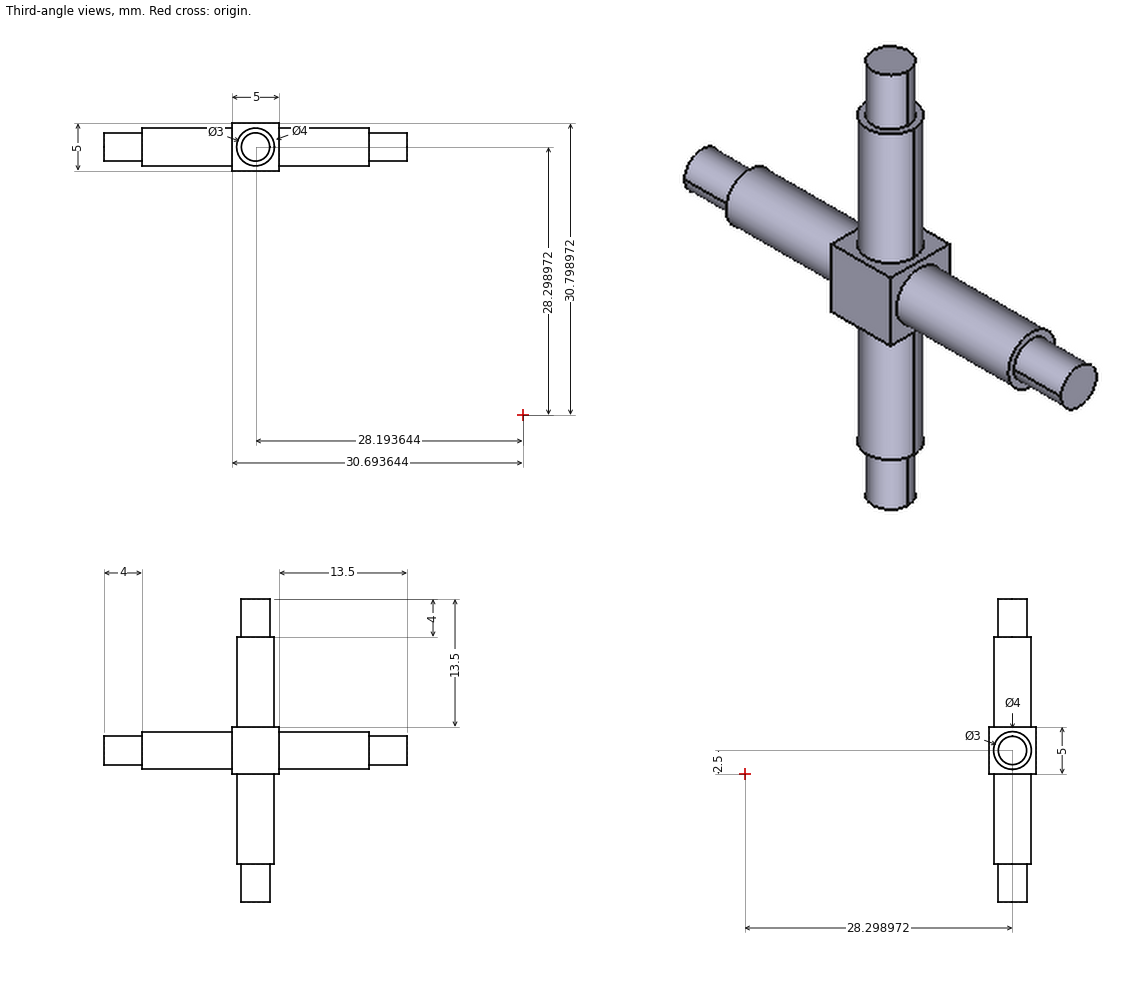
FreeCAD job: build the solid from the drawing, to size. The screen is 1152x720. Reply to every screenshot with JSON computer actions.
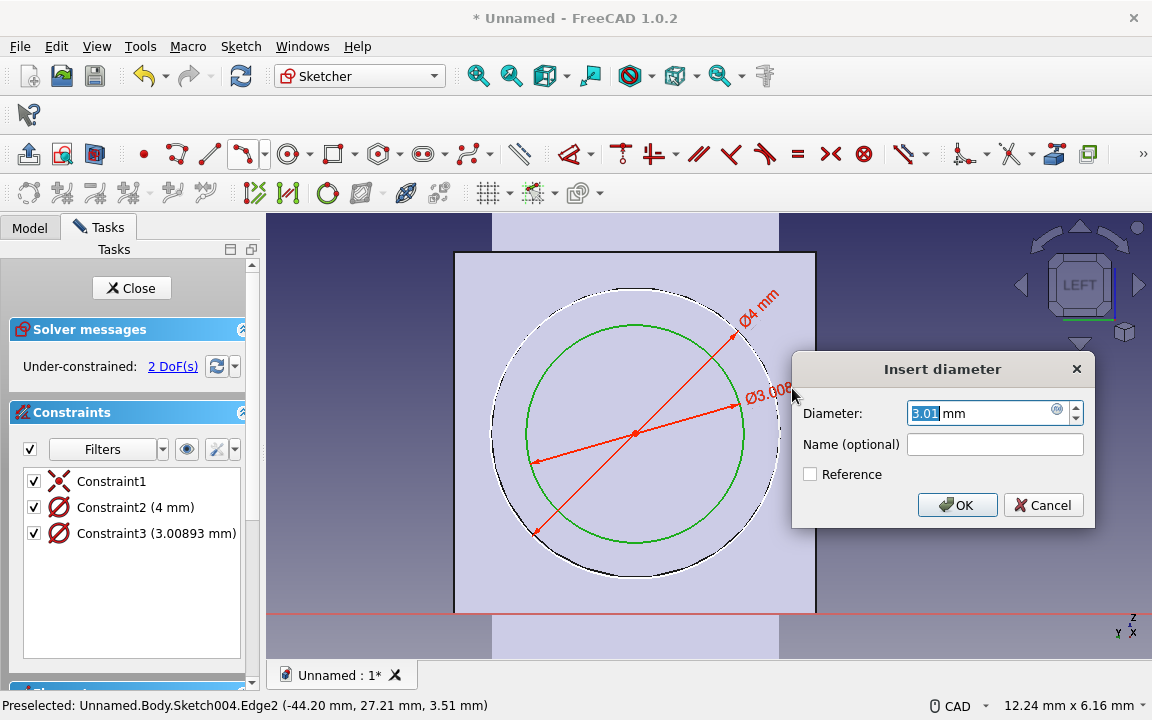
{"action": "type", "text": "3"}
{"action": "key", "text": "Return"}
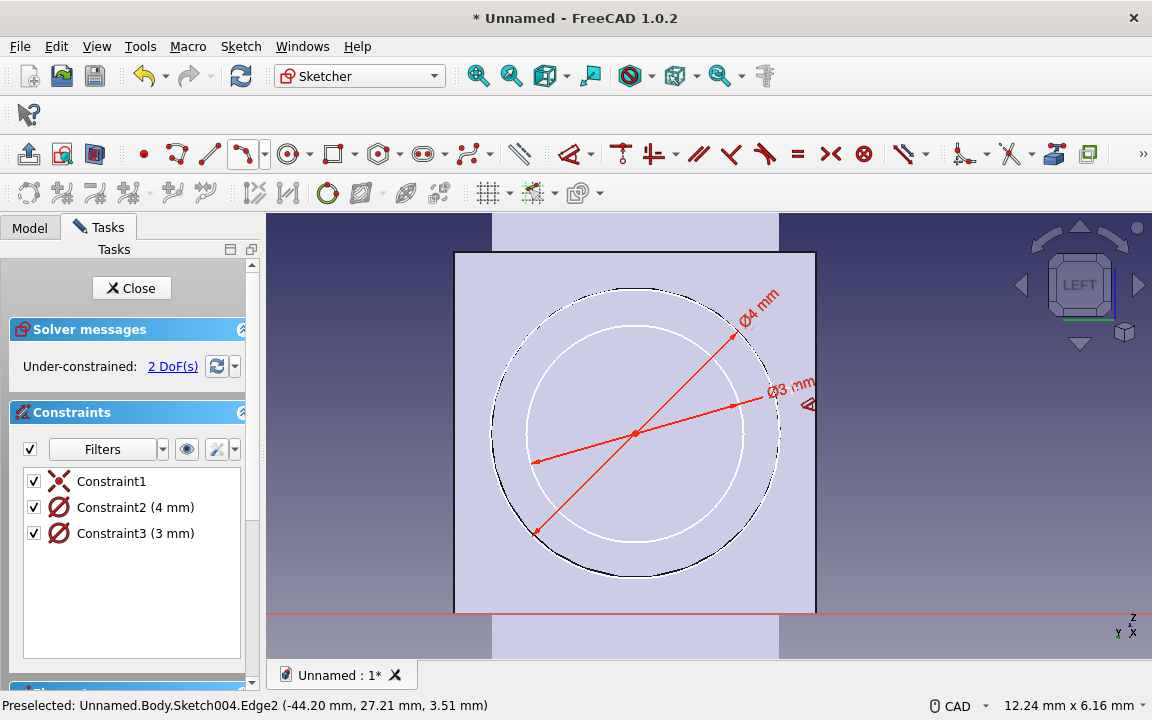
{"action": "left_click", "coordinate": [635, 434]}
{"action": "left_click", "coordinate": [601, 483]}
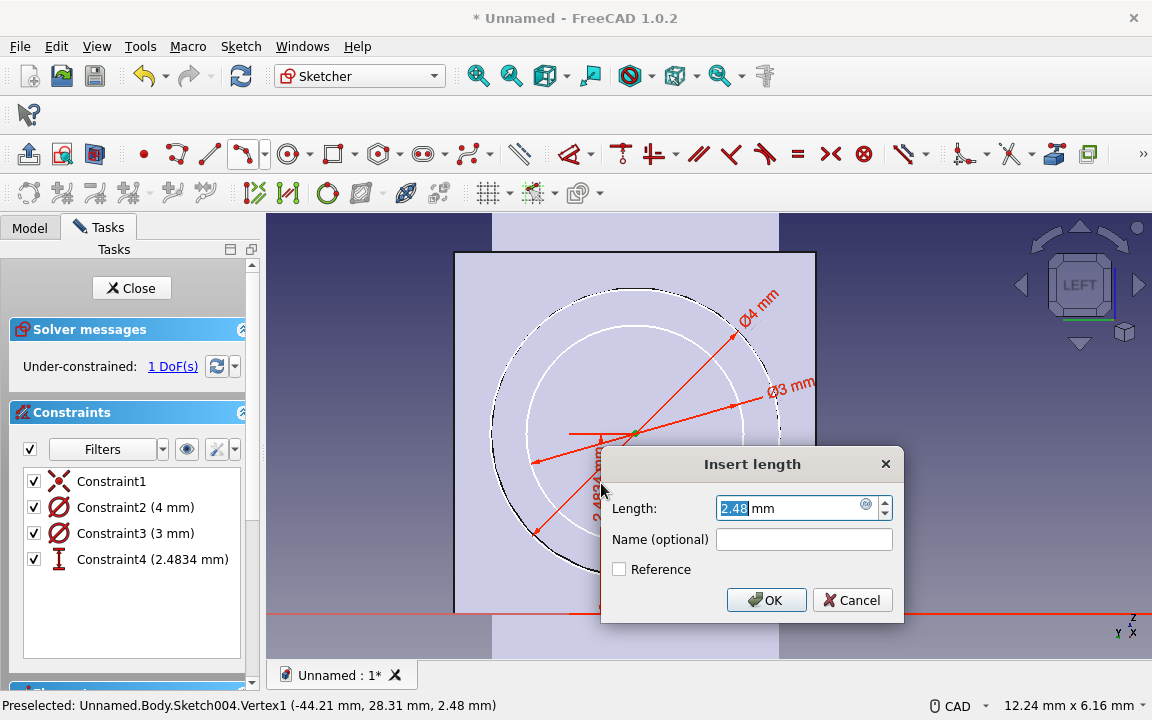
{"action": "type", "text": "2.5"}
{"action": "key", "text": "Return"}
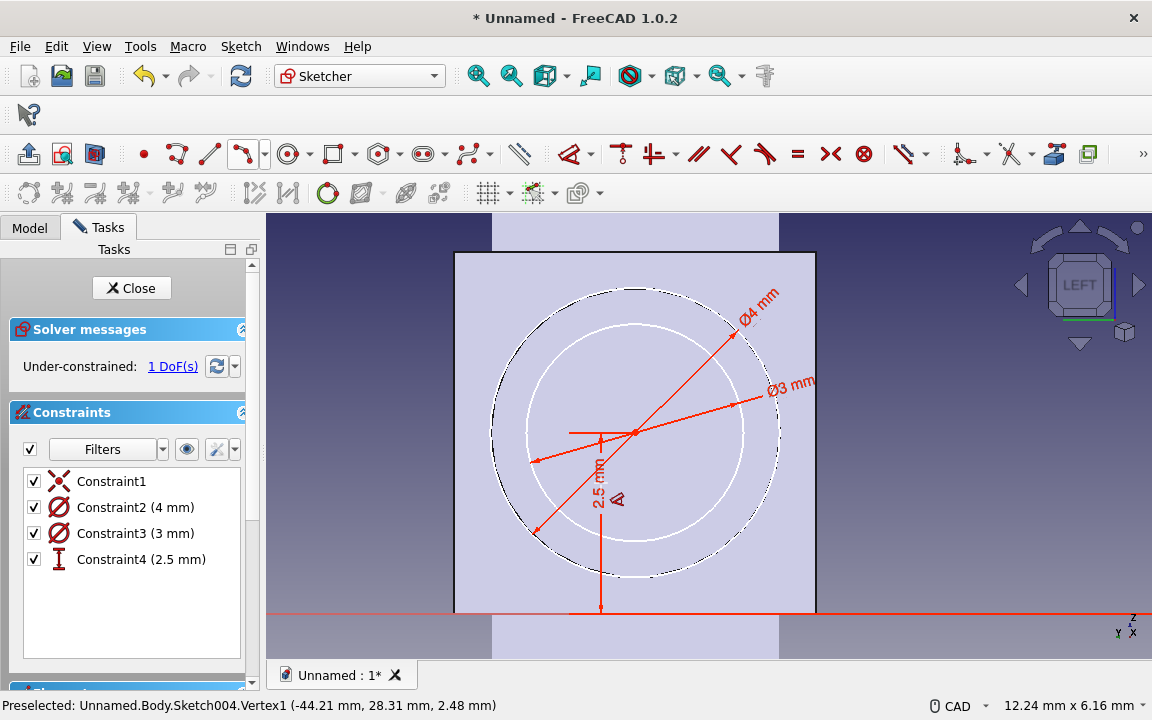
{"action": "left_click", "coordinate": [635, 433]}
{"action": "left_click", "coordinate": [892, 399]}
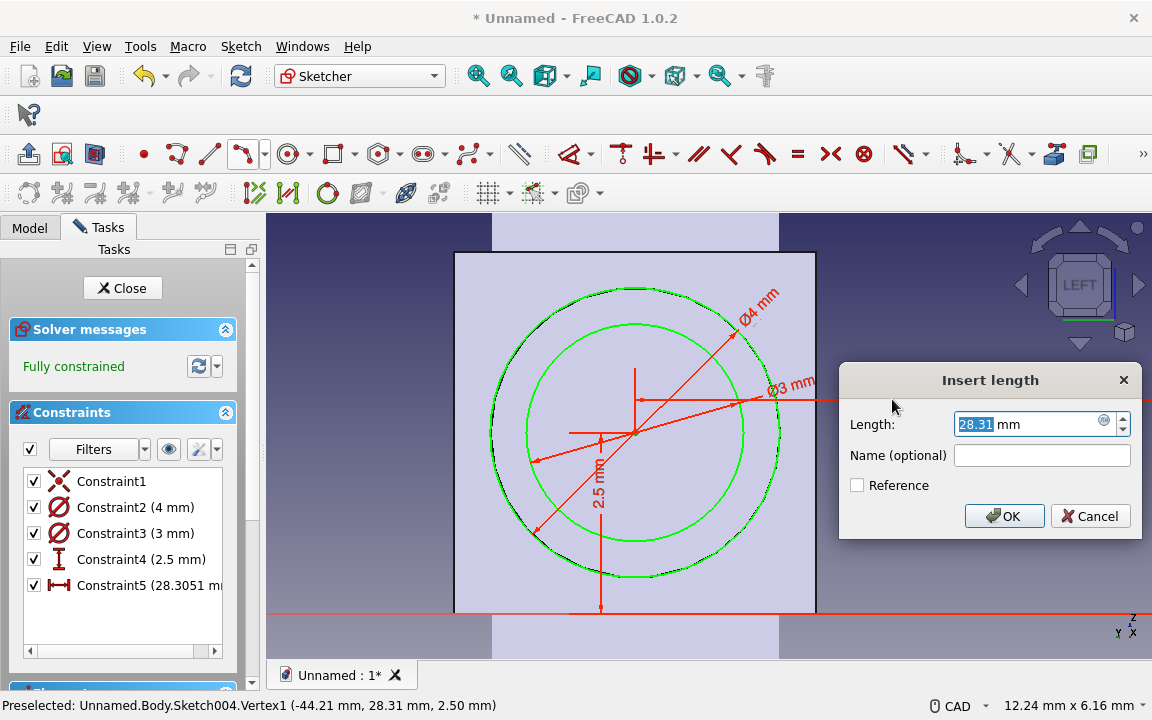
{"action": "type", "text": "28.298972"}
{"action": "key", "text": "Return"}
{"action": "key", "text": "Escape"}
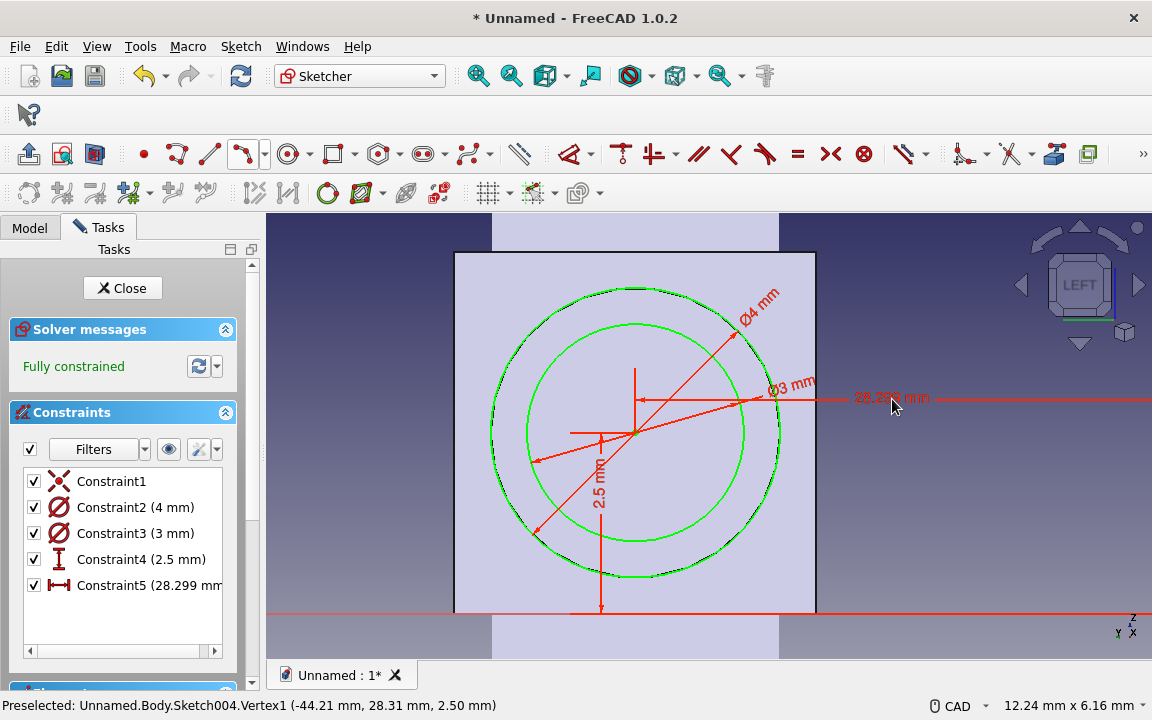
{"action": "left_click", "coordinate": [123, 288]}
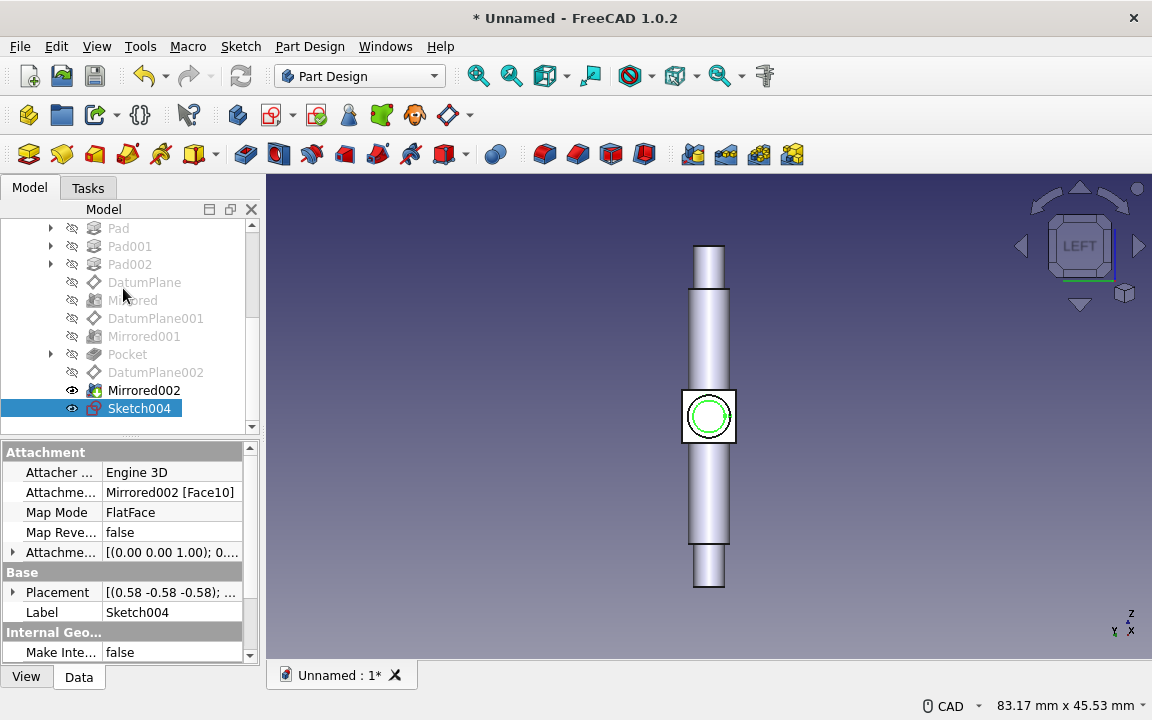
{"action": "left_click", "coordinate": [246, 154]}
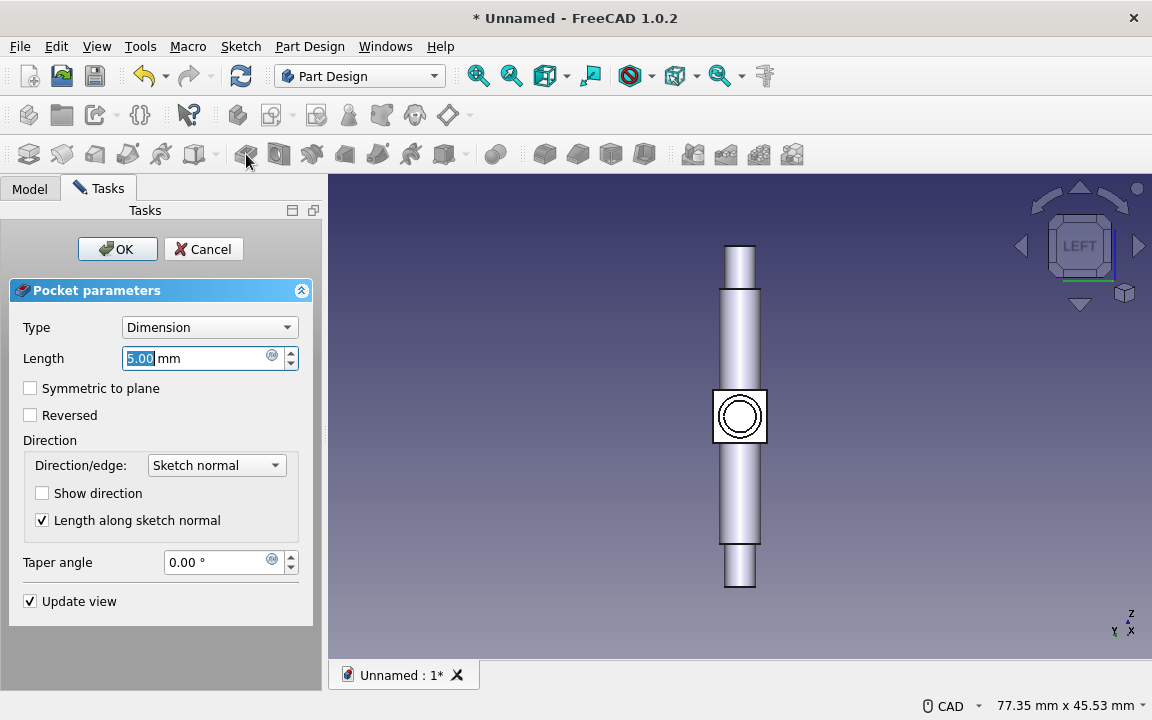
{"action": "type", "text": "4"}
{"action": "key", "text": "Tab"}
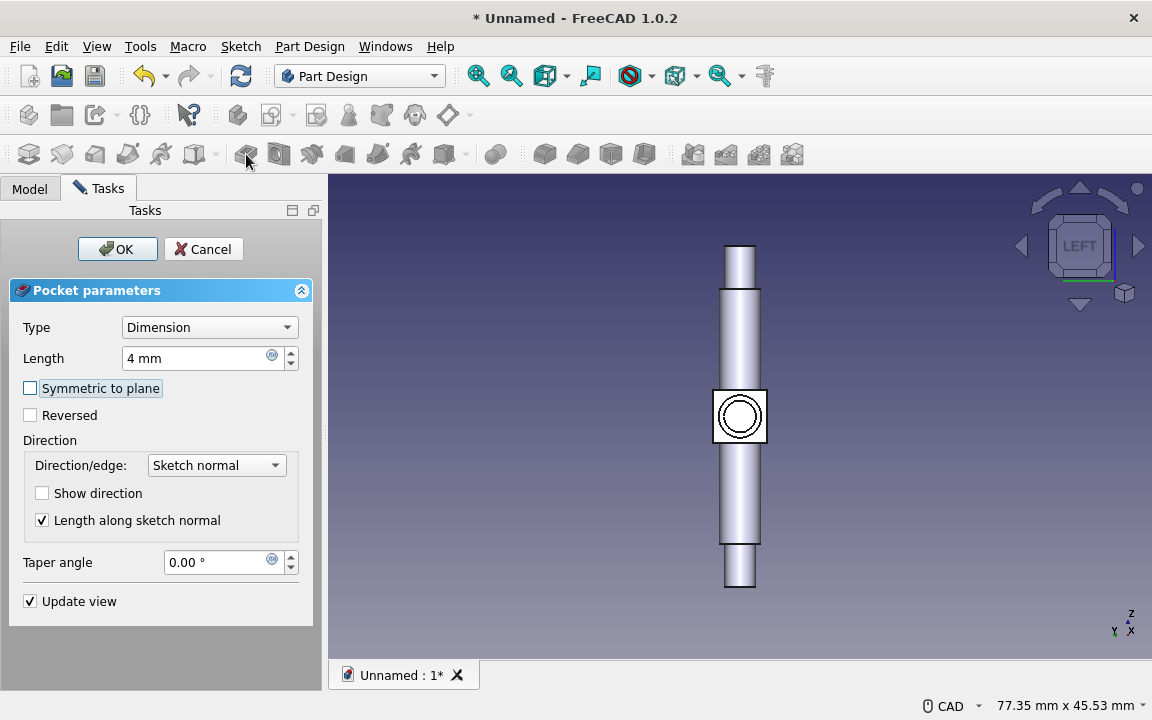
{"action": "left_click", "coordinate": [118, 249]}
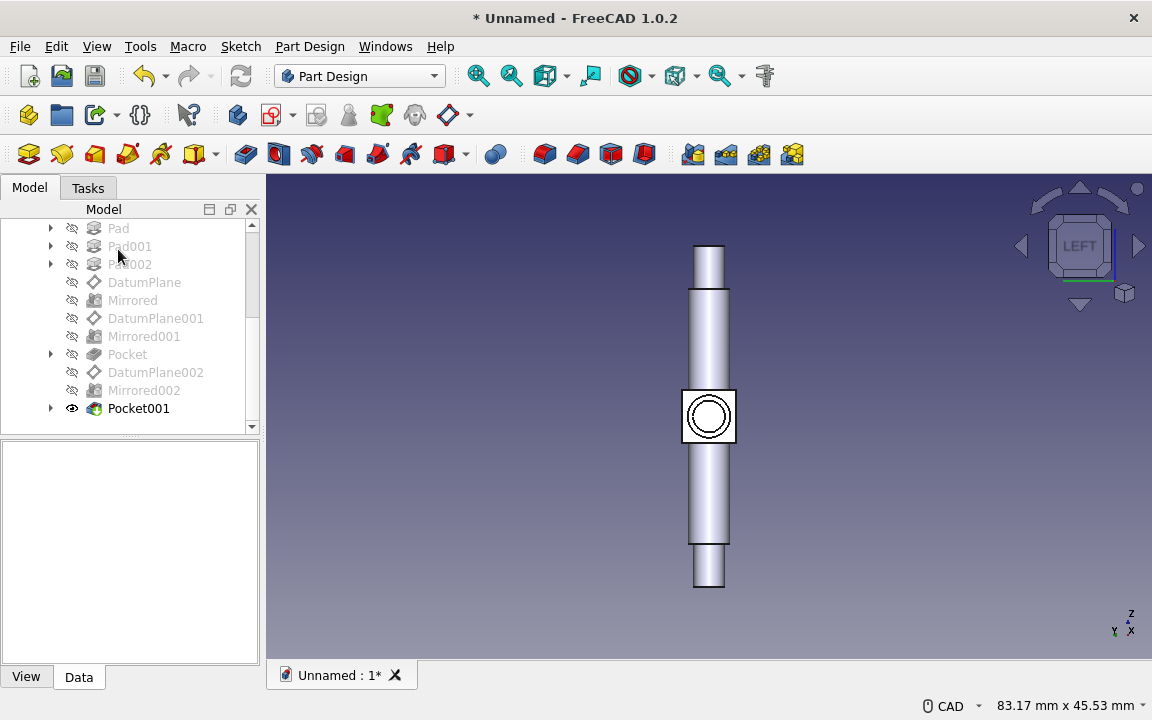
{"action": "scroll", "coordinate": [141, 314], "scroll_direction": "down", "scroll_amount": 3}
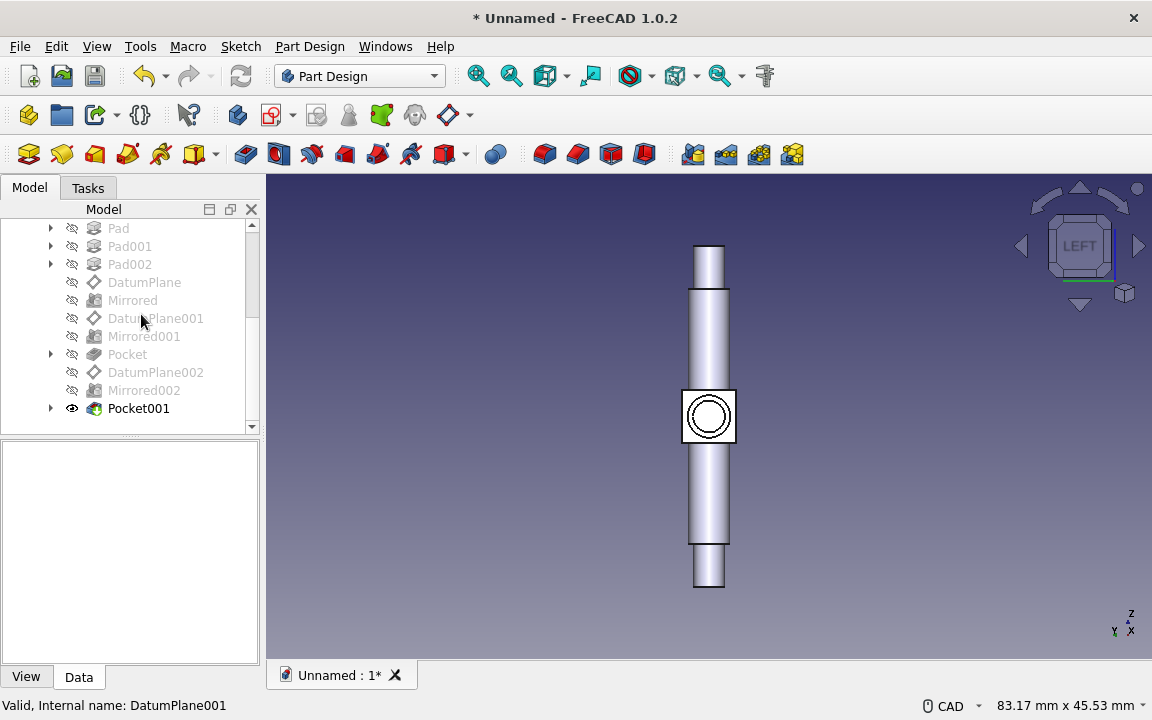
{"action": "scroll", "coordinate": [141, 314], "scroll_direction": "up", "scroll_amount": 15}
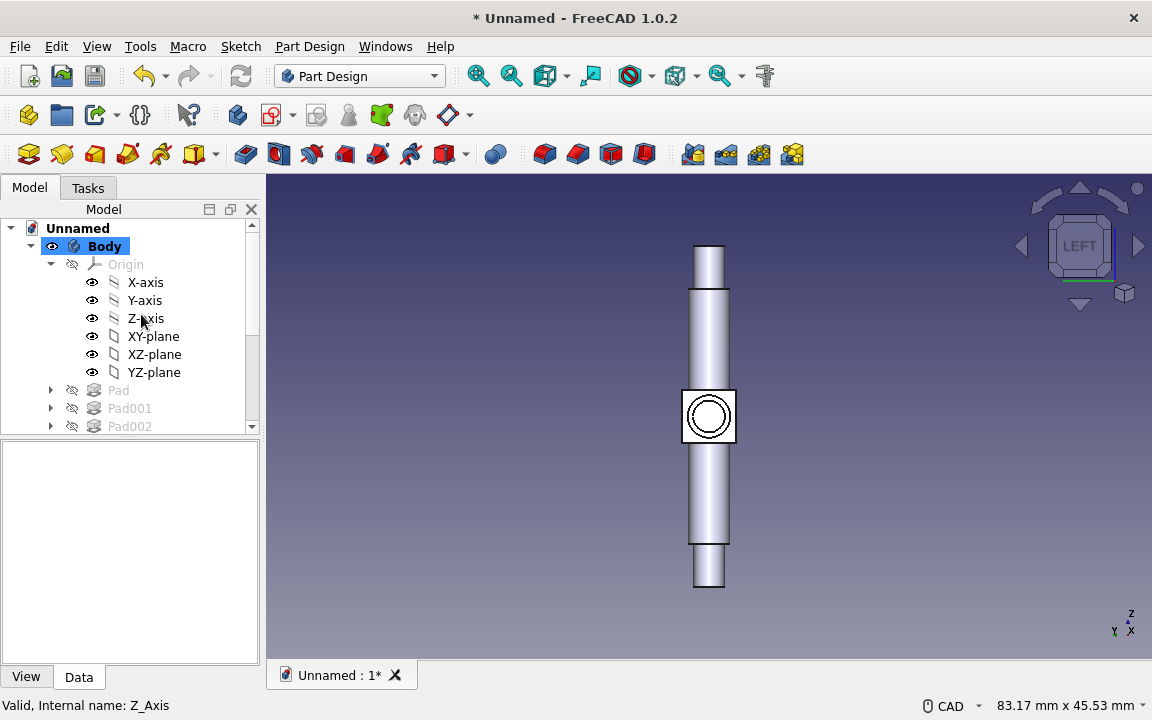
{"action": "left_click", "coordinate": [137, 372]}